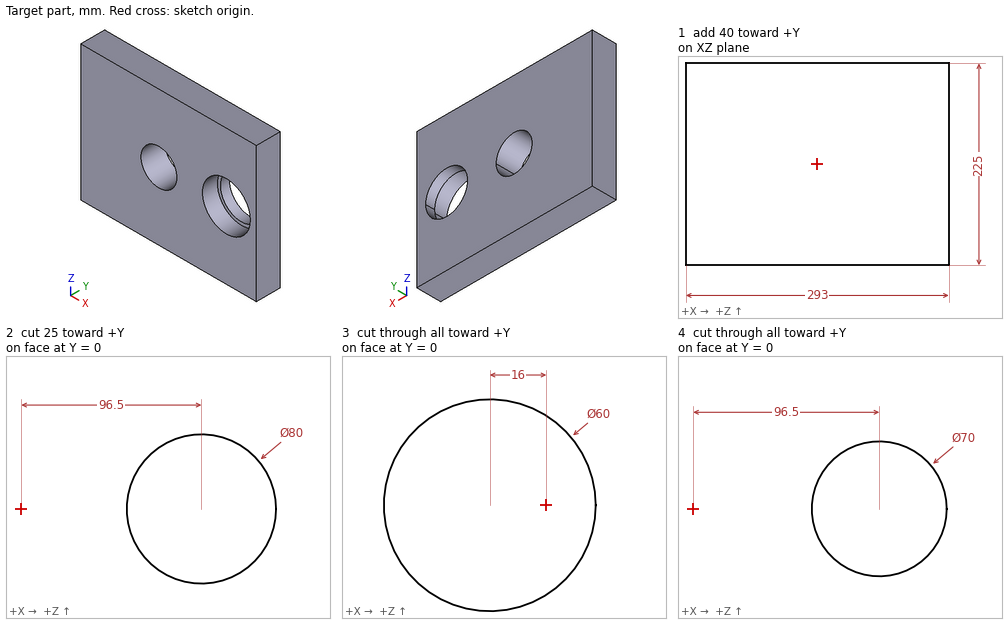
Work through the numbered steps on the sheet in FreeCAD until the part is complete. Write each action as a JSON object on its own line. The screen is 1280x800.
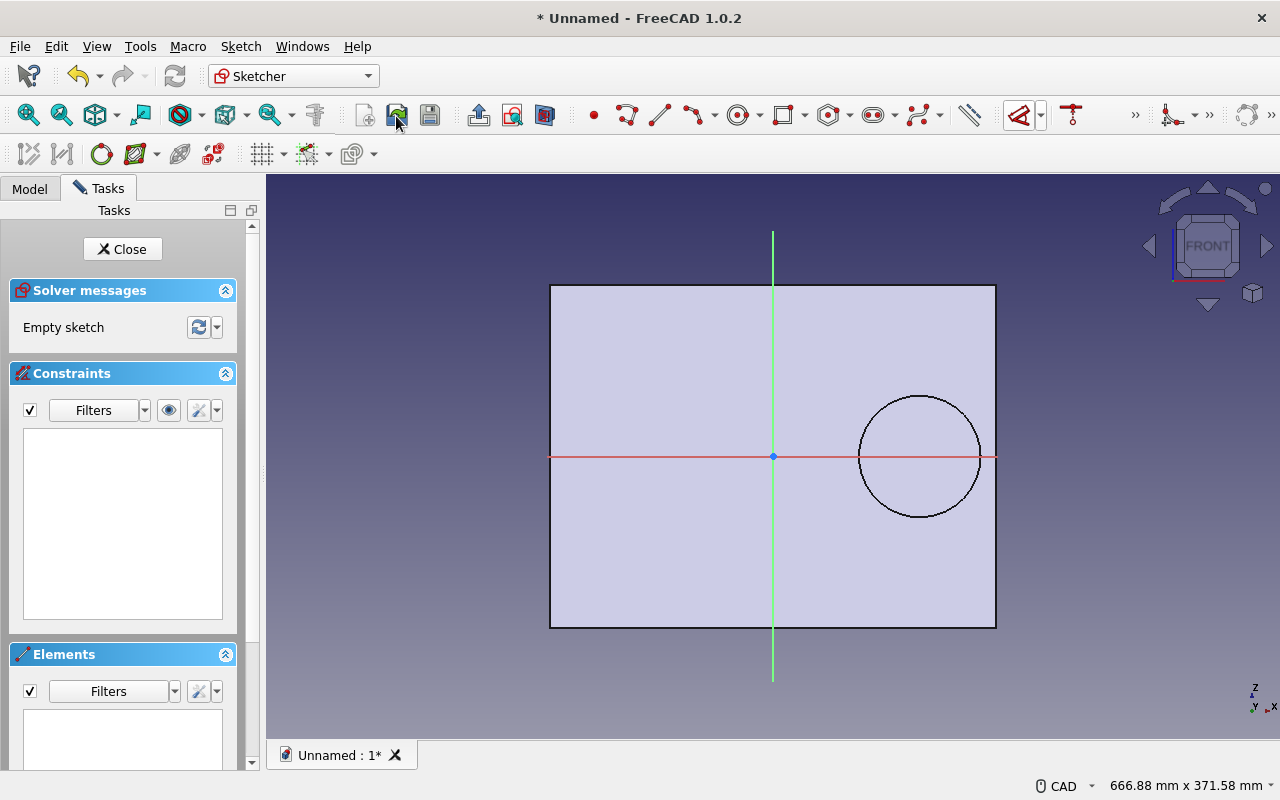
{"action": "scroll", "coordinate": [763, 457], "scroll_direction": "up", "scroll_amount": 7}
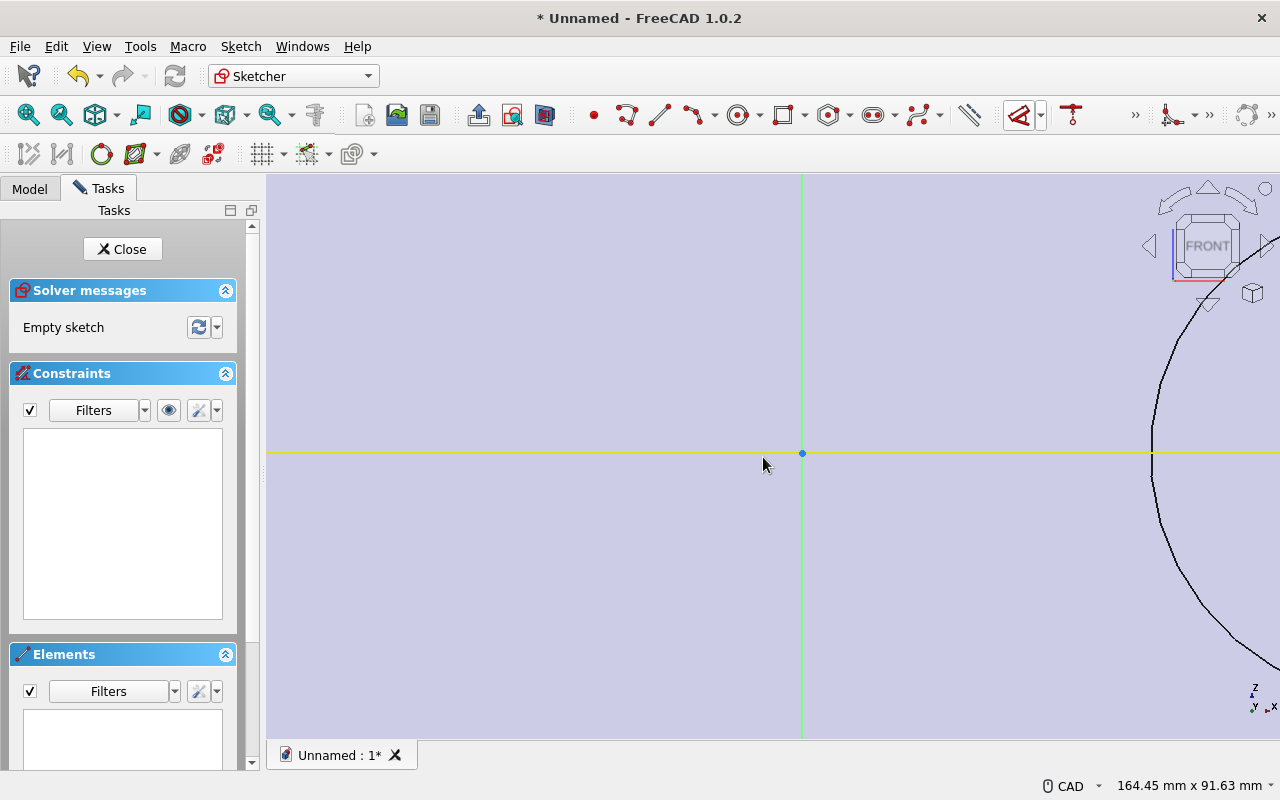
{"action": "left_click", "coordinate": [738, 116]}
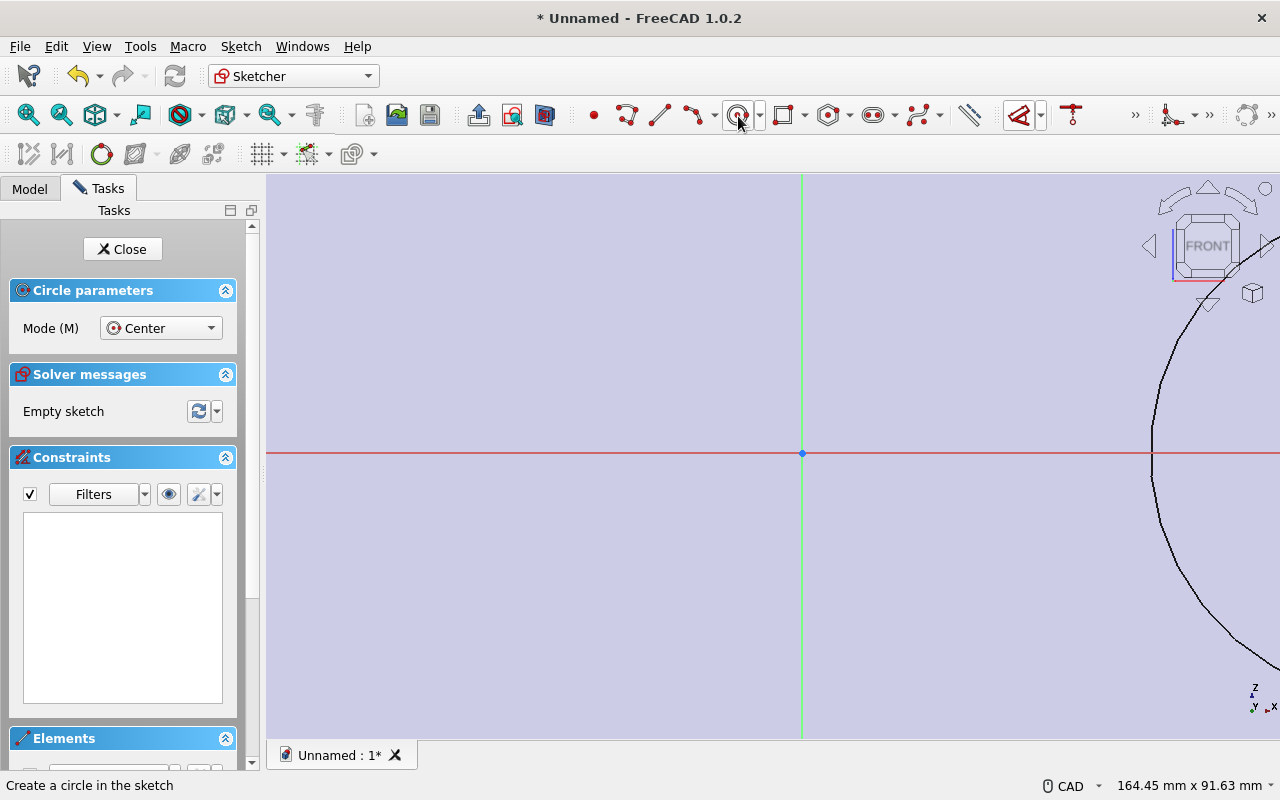
{"action": "left_click", "coordinate": [703, 453]}
{"action": "mouse_move", "coordinate": [834, 323]}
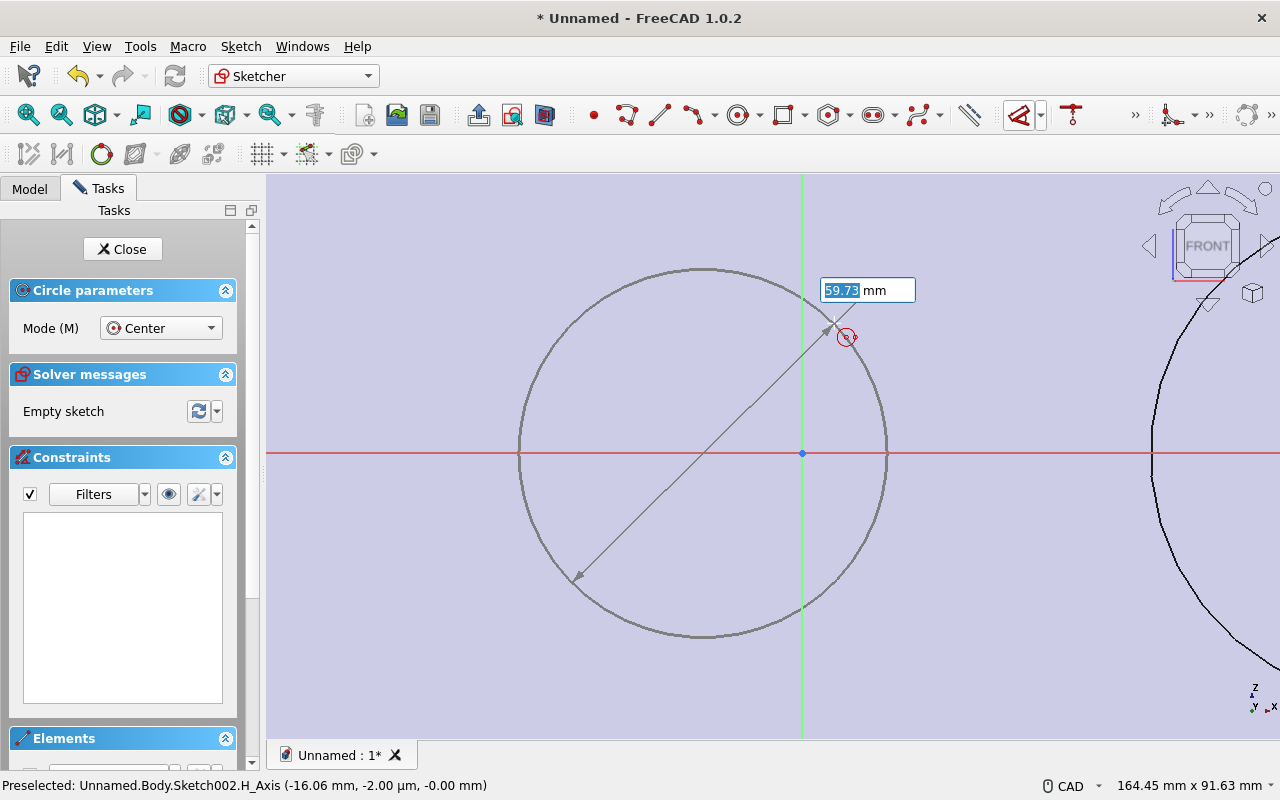
{"action": "type", "text": "60"}
{"action": "key", "text": "Return"}
{"action": "key", "text": "Escape"}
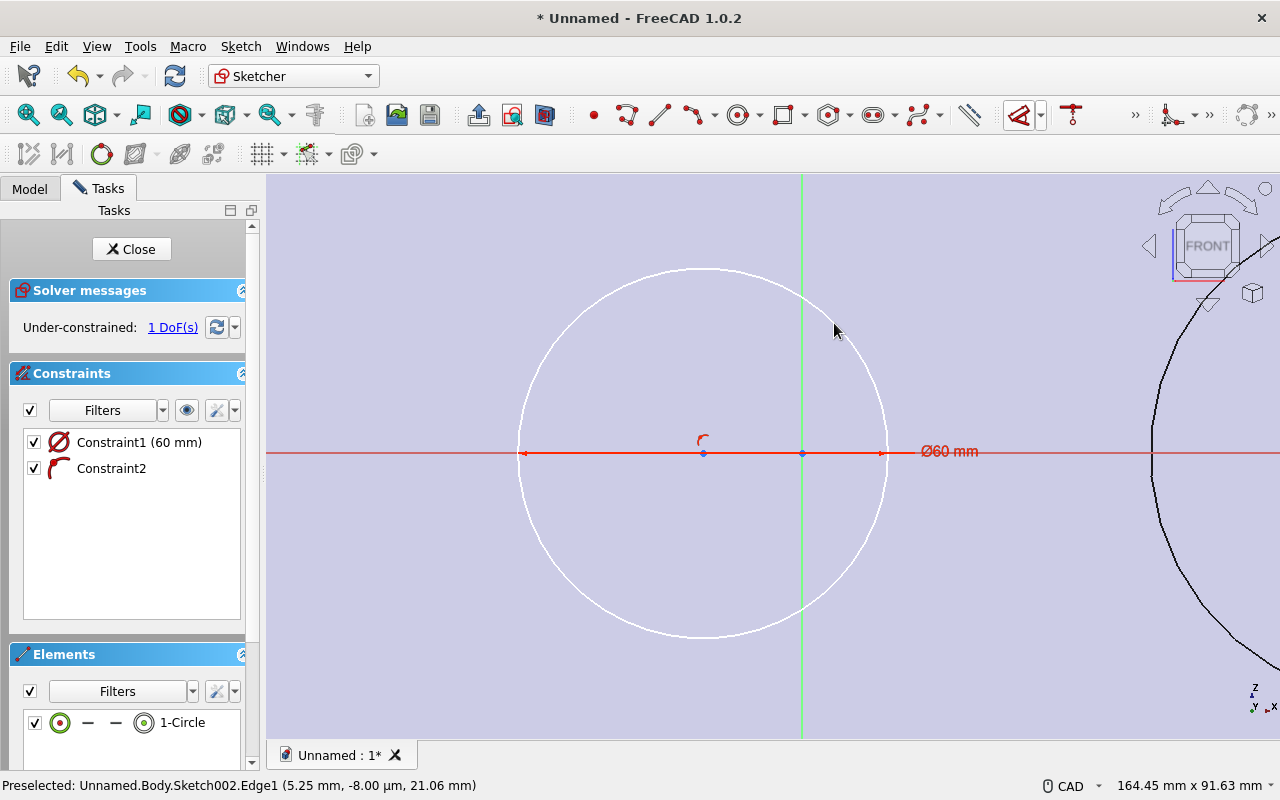
{"action": "left_click", "coordinate": [703, 453]}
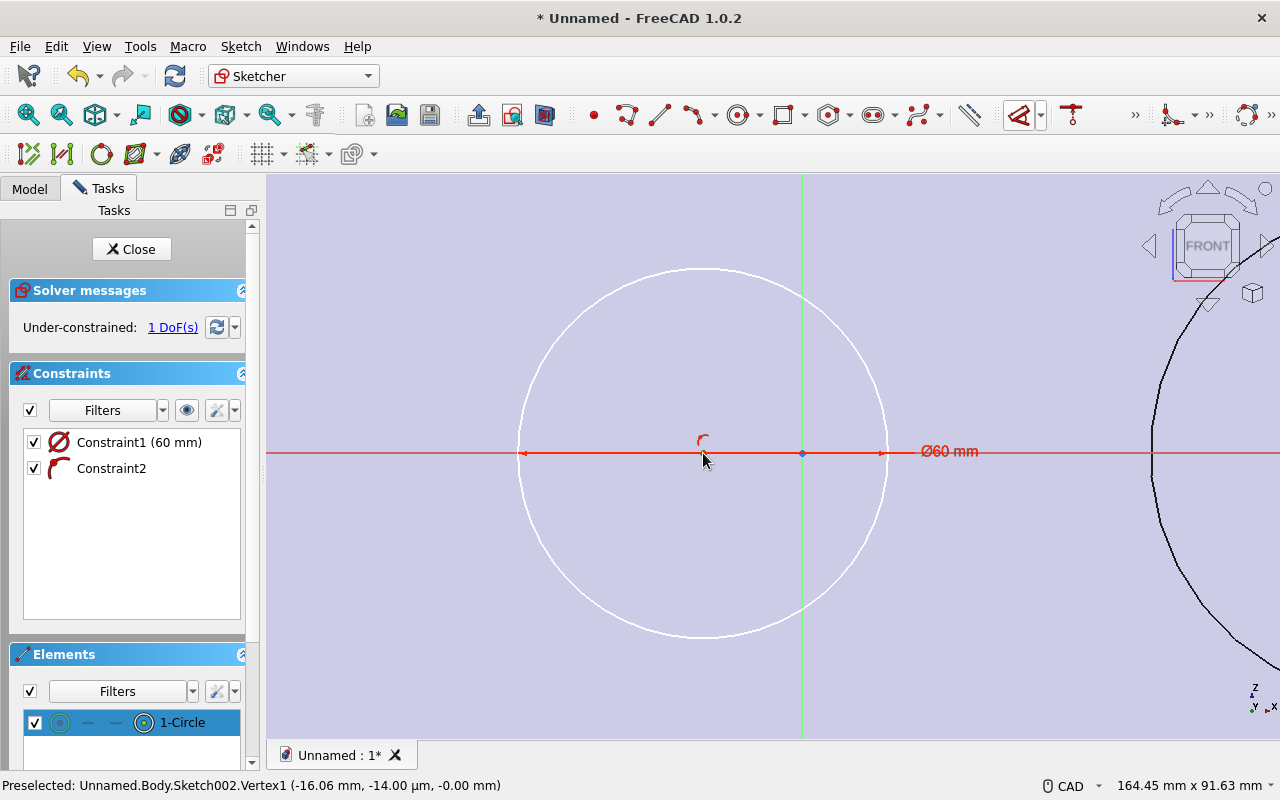
{"action": "left_click", "coordinate": [1040, 116]}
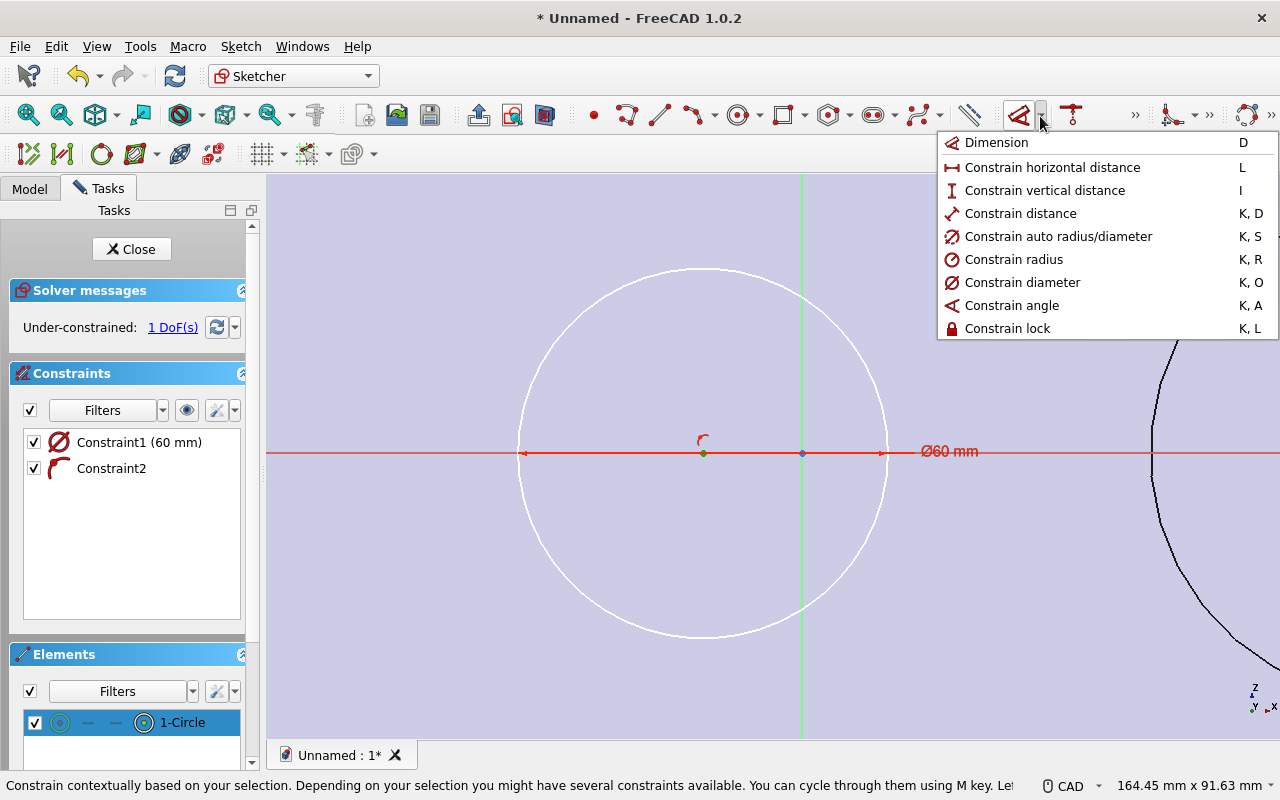
{"action": "left_click", "coordinate": [1108, 168]}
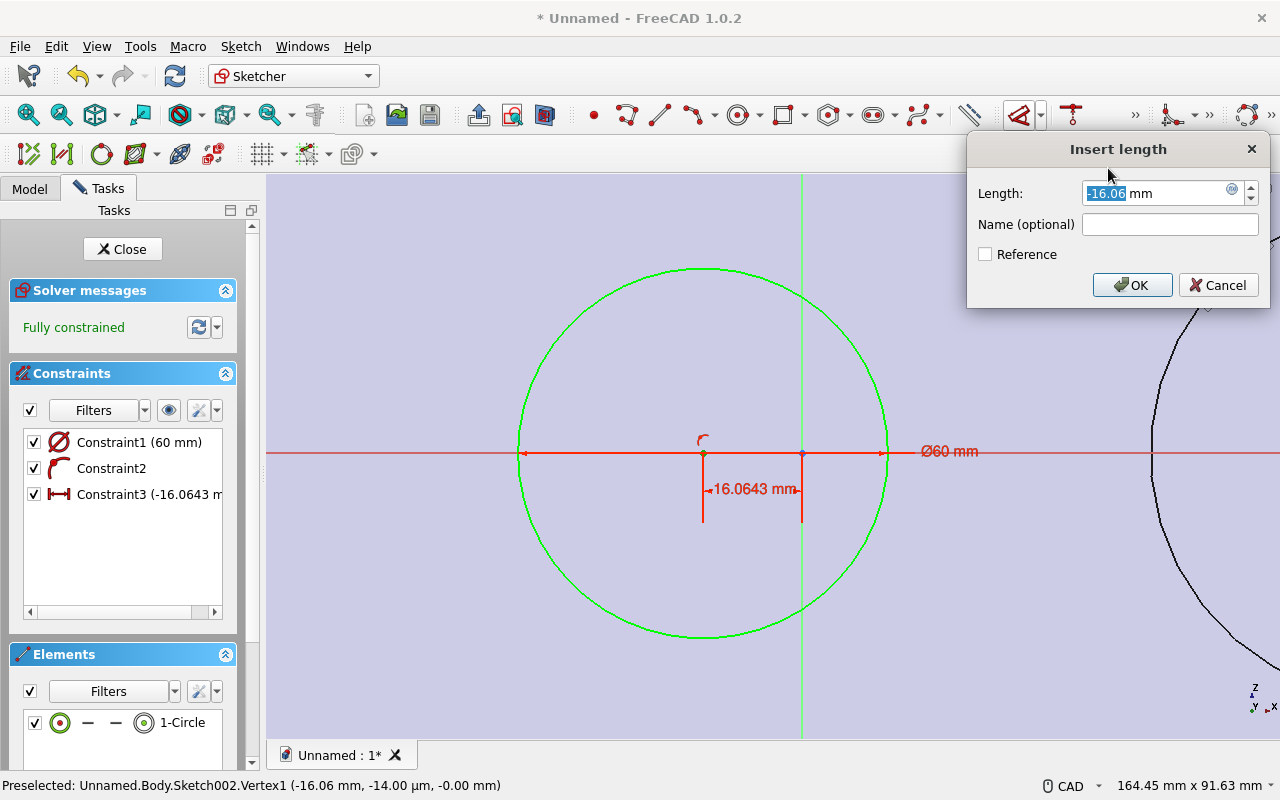
{"action": "type", "text": "-16"}
{"action": "key", "text": "Return"}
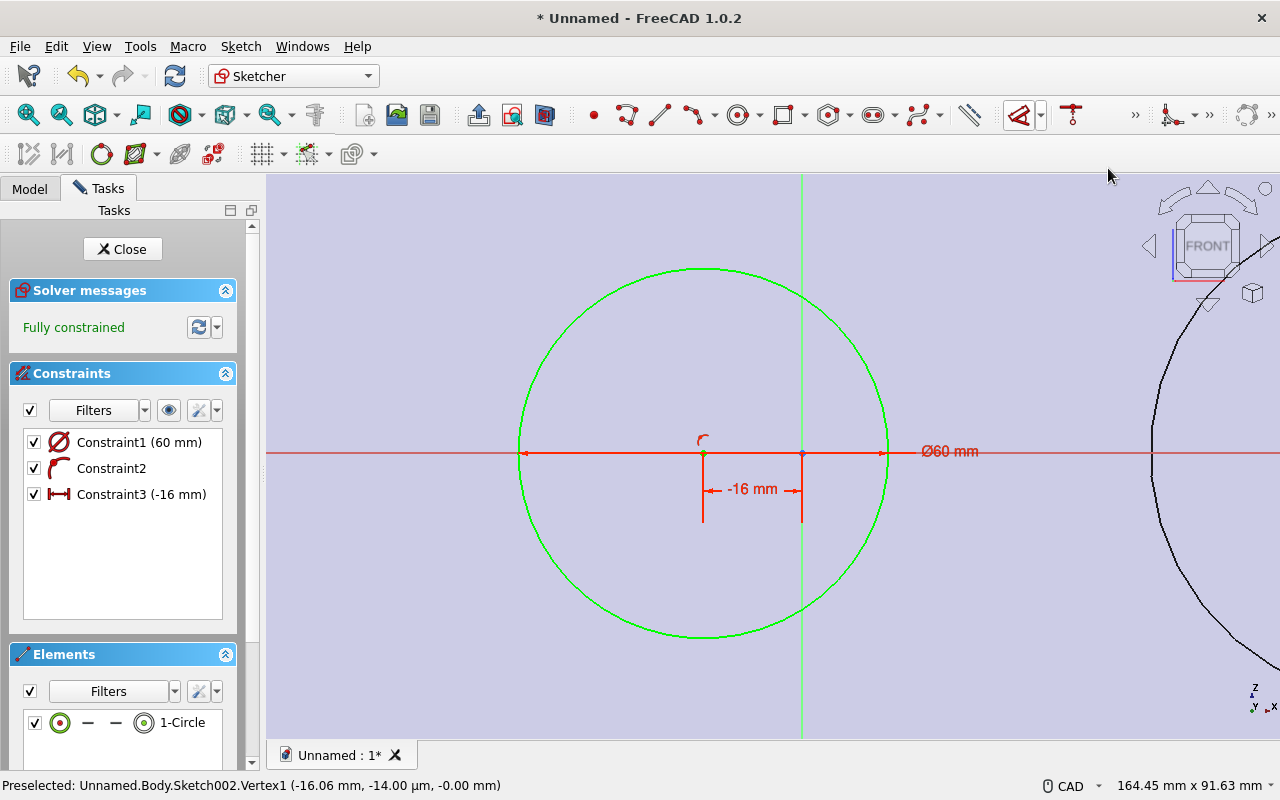
{"action": "left_click", "coordinate": [123, 249]}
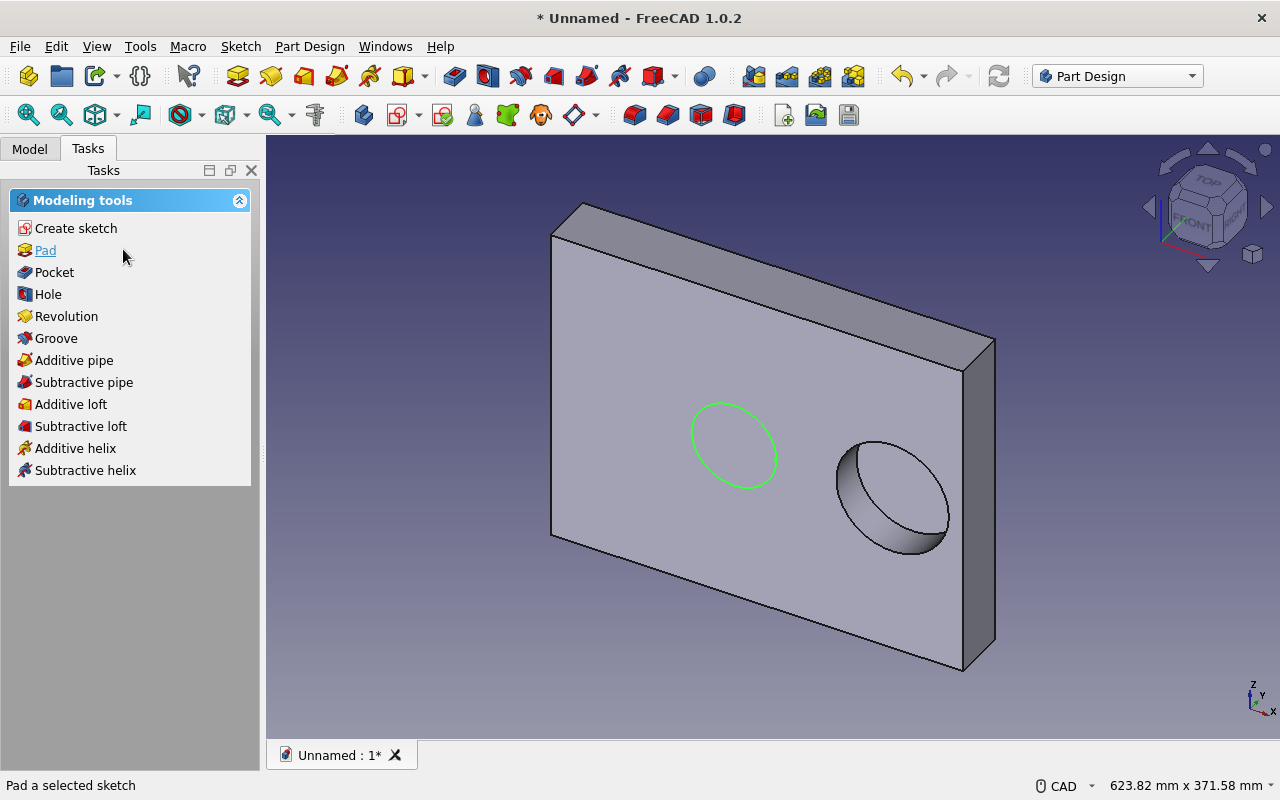
{"action": "left_click", "coordinate": [455, 76]}